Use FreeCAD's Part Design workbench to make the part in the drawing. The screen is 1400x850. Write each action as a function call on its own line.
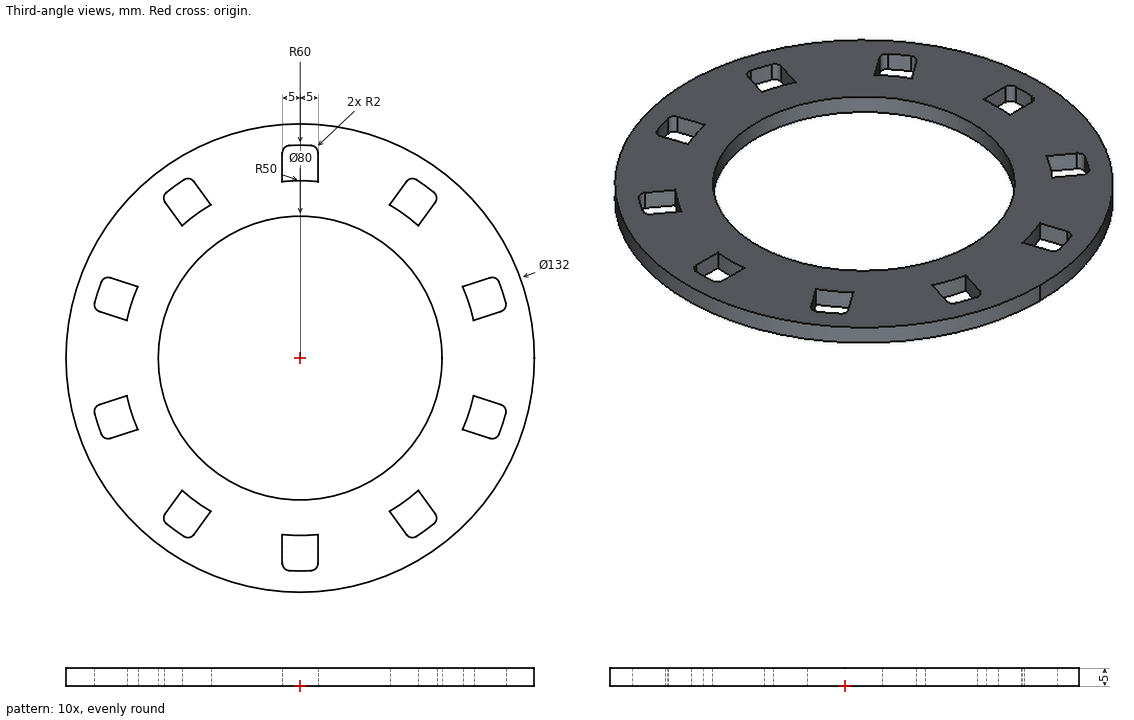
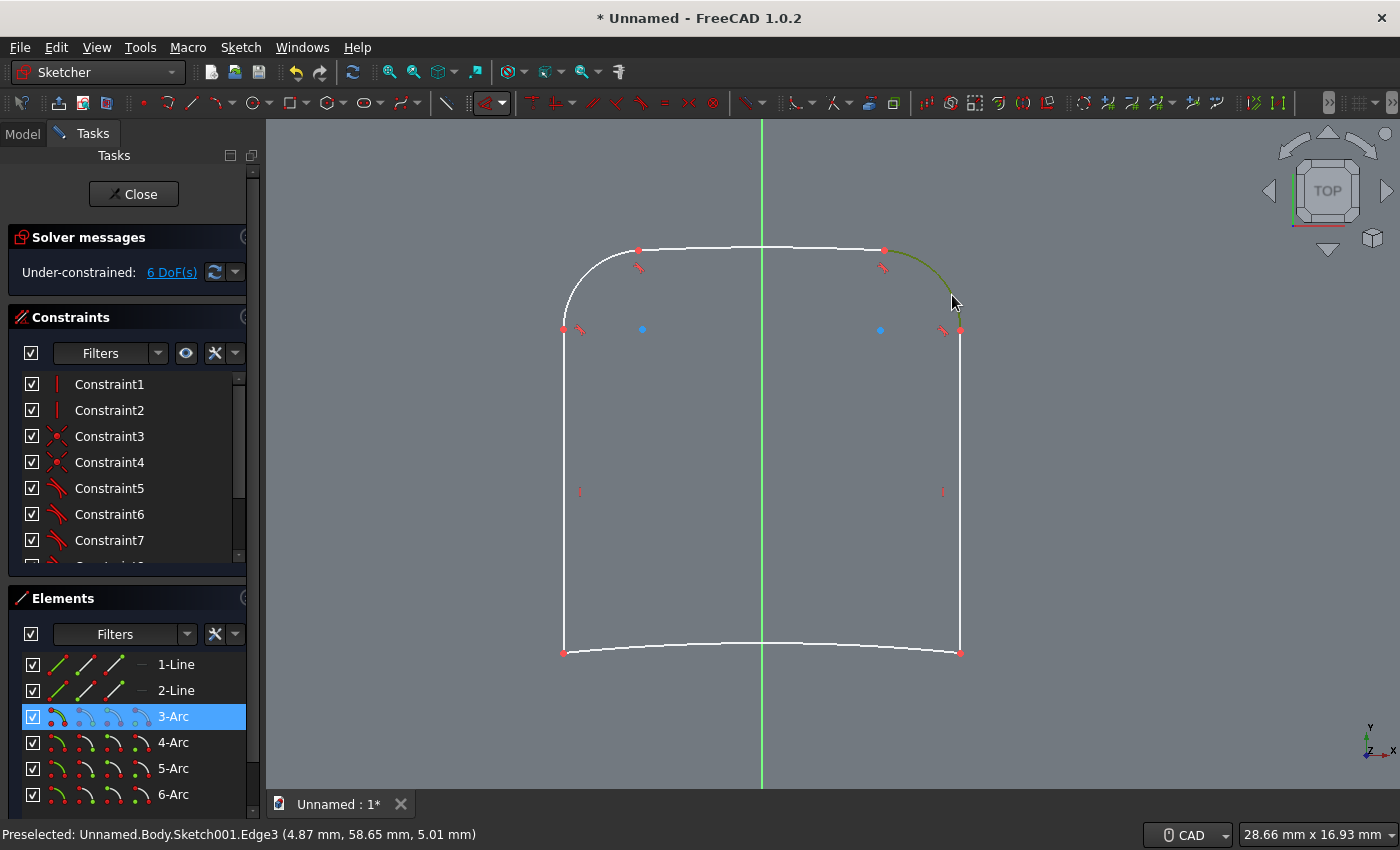
click(604, 260)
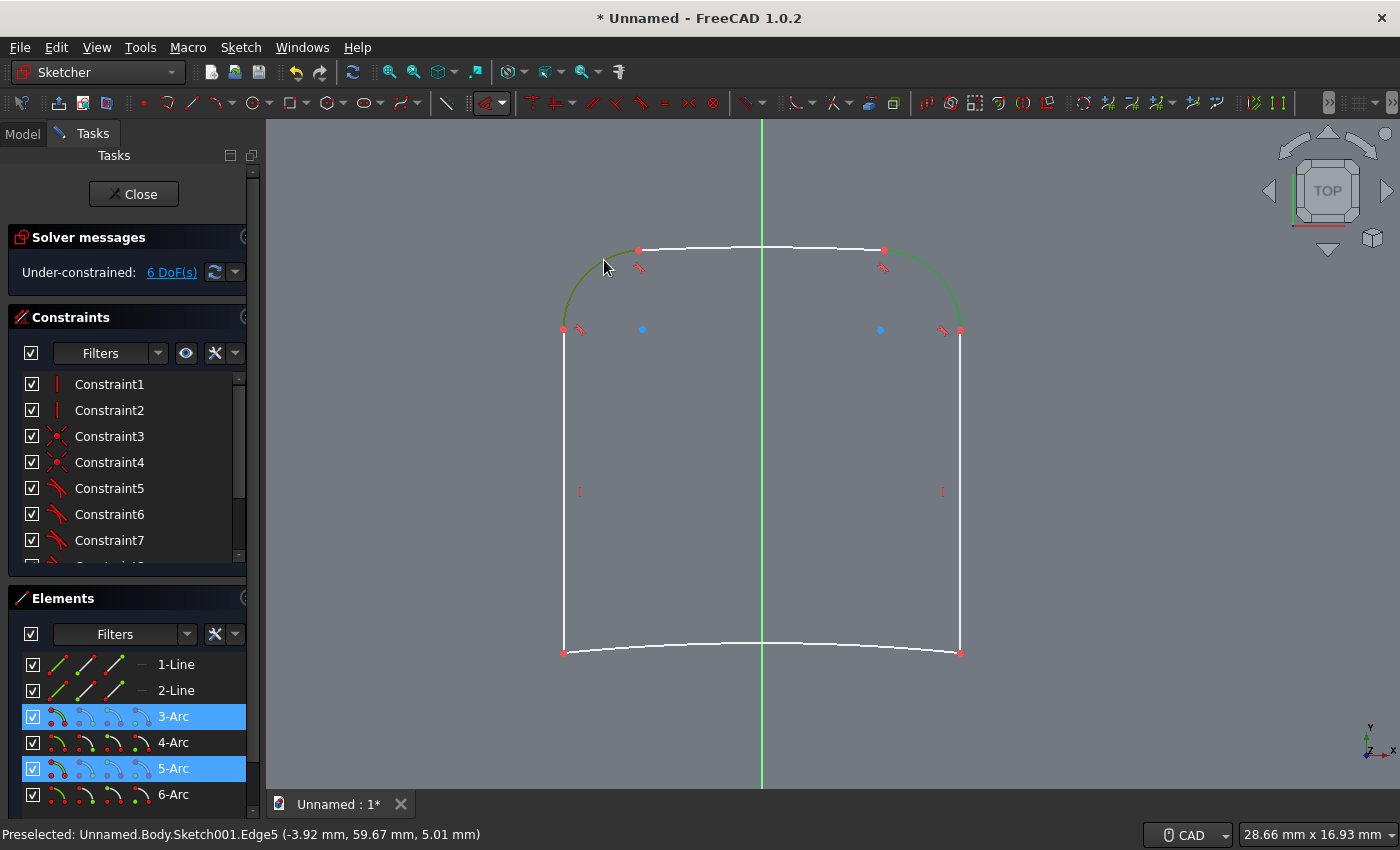
key(e)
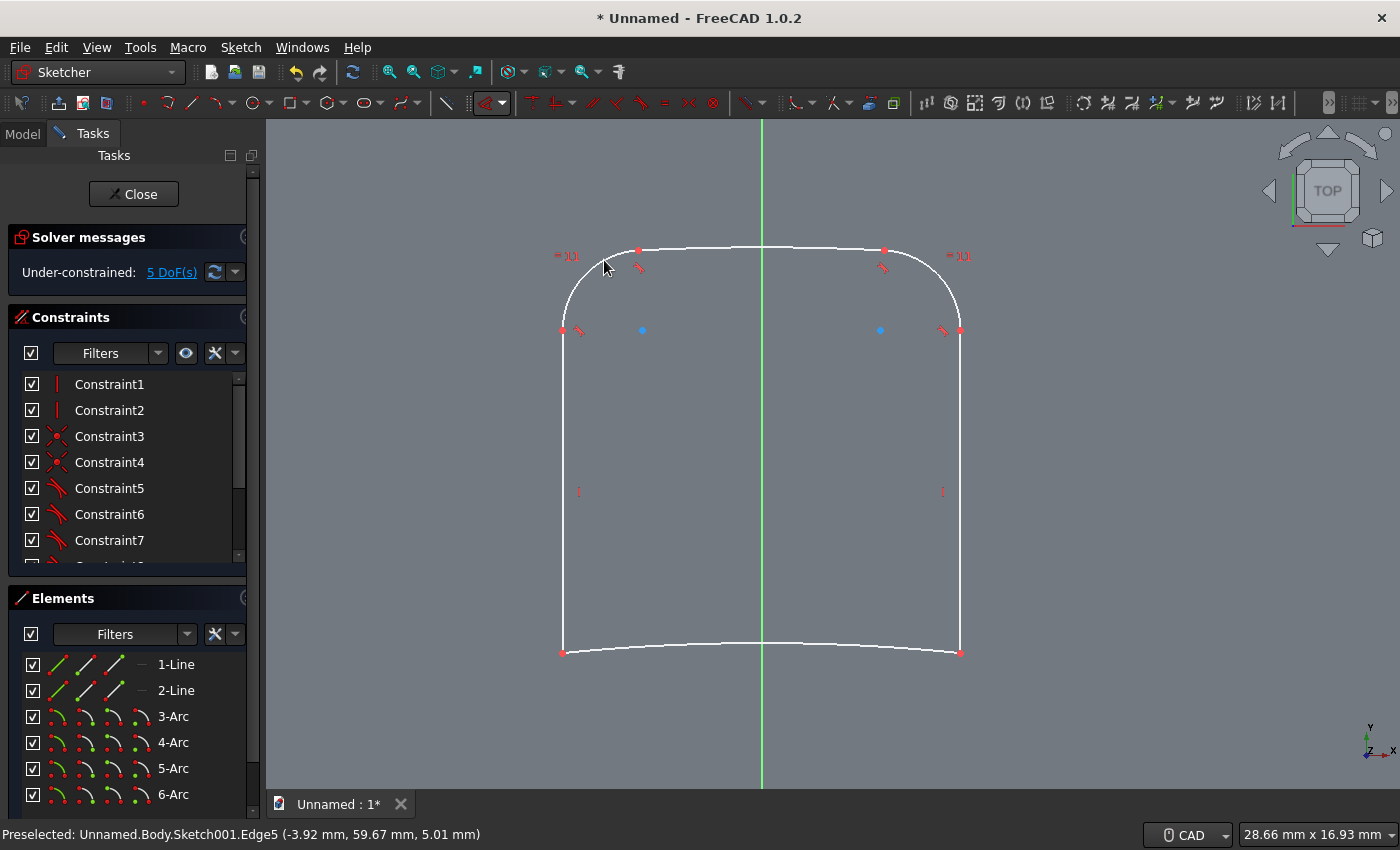
key(d)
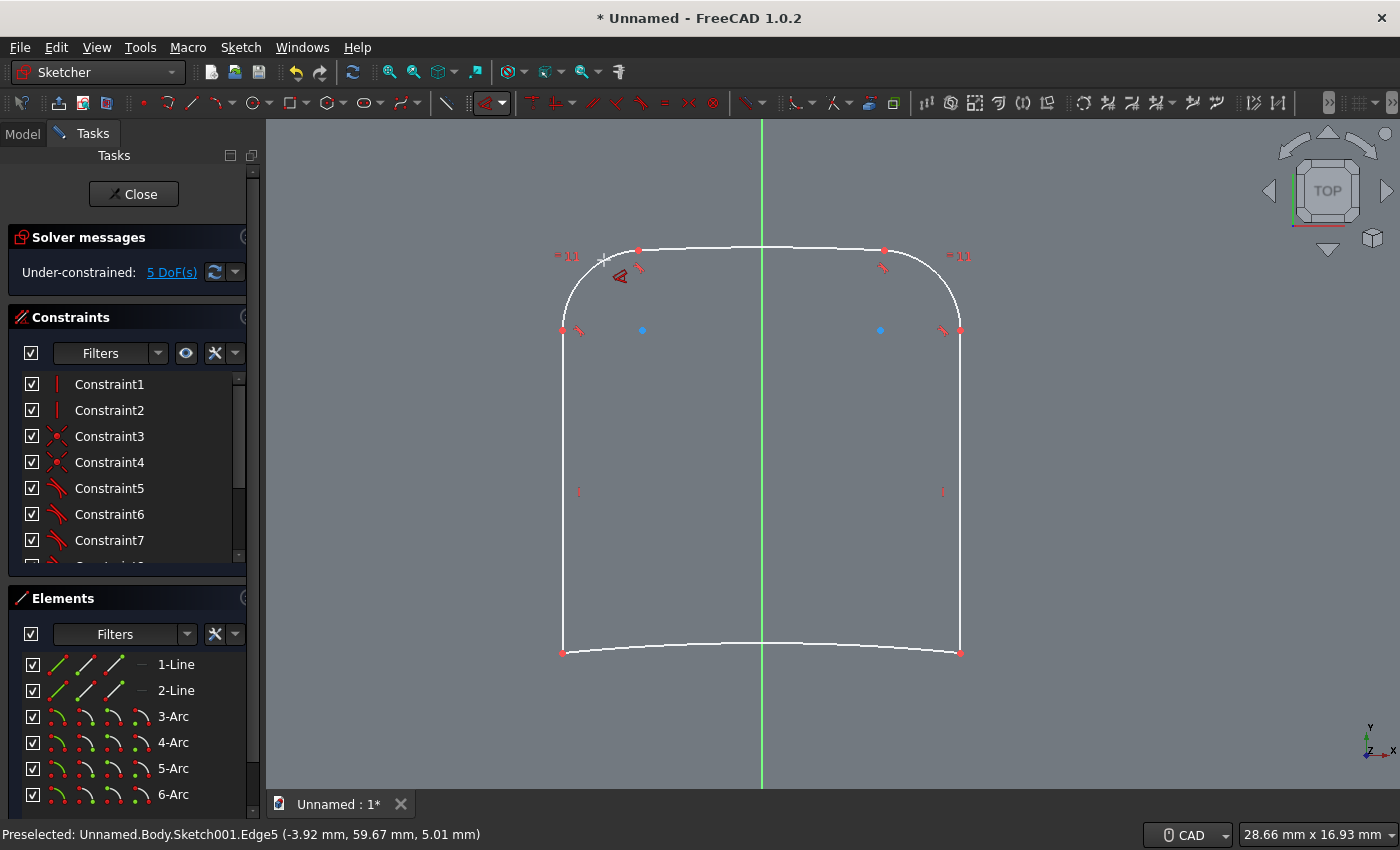
click(952, 295)
click(981, 281)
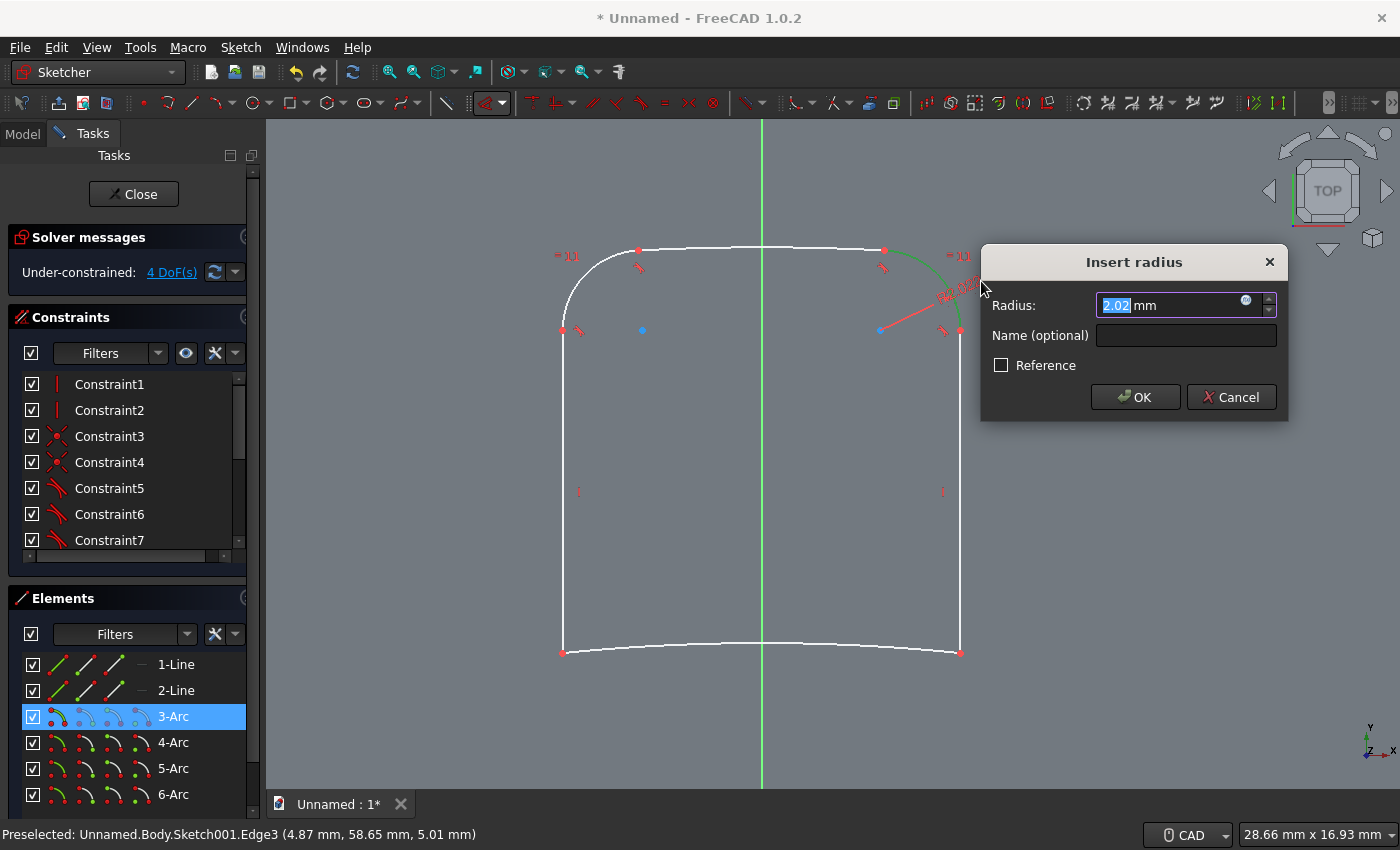
text(2)
key(Return)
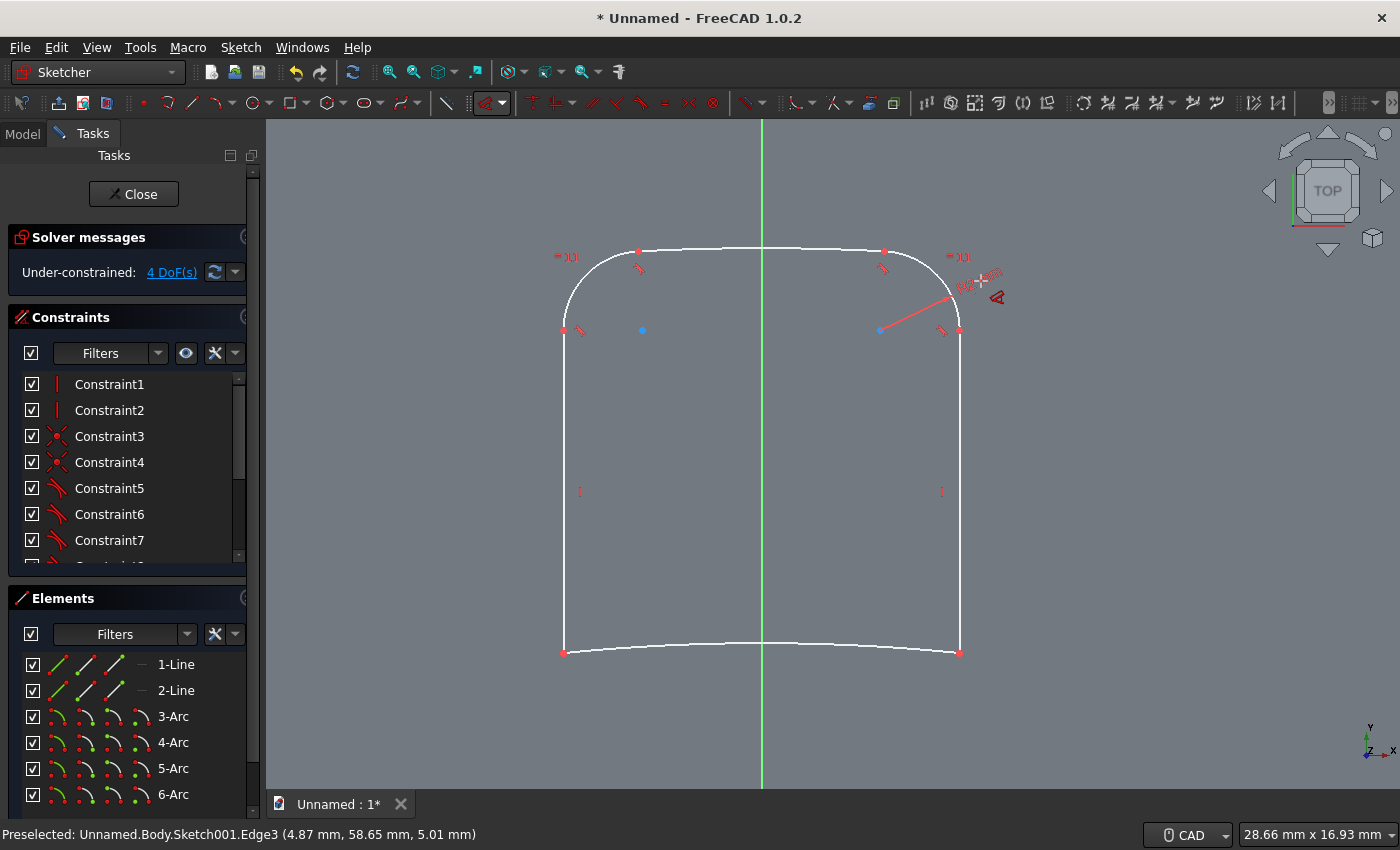
click(811, 249)
click(812, 217)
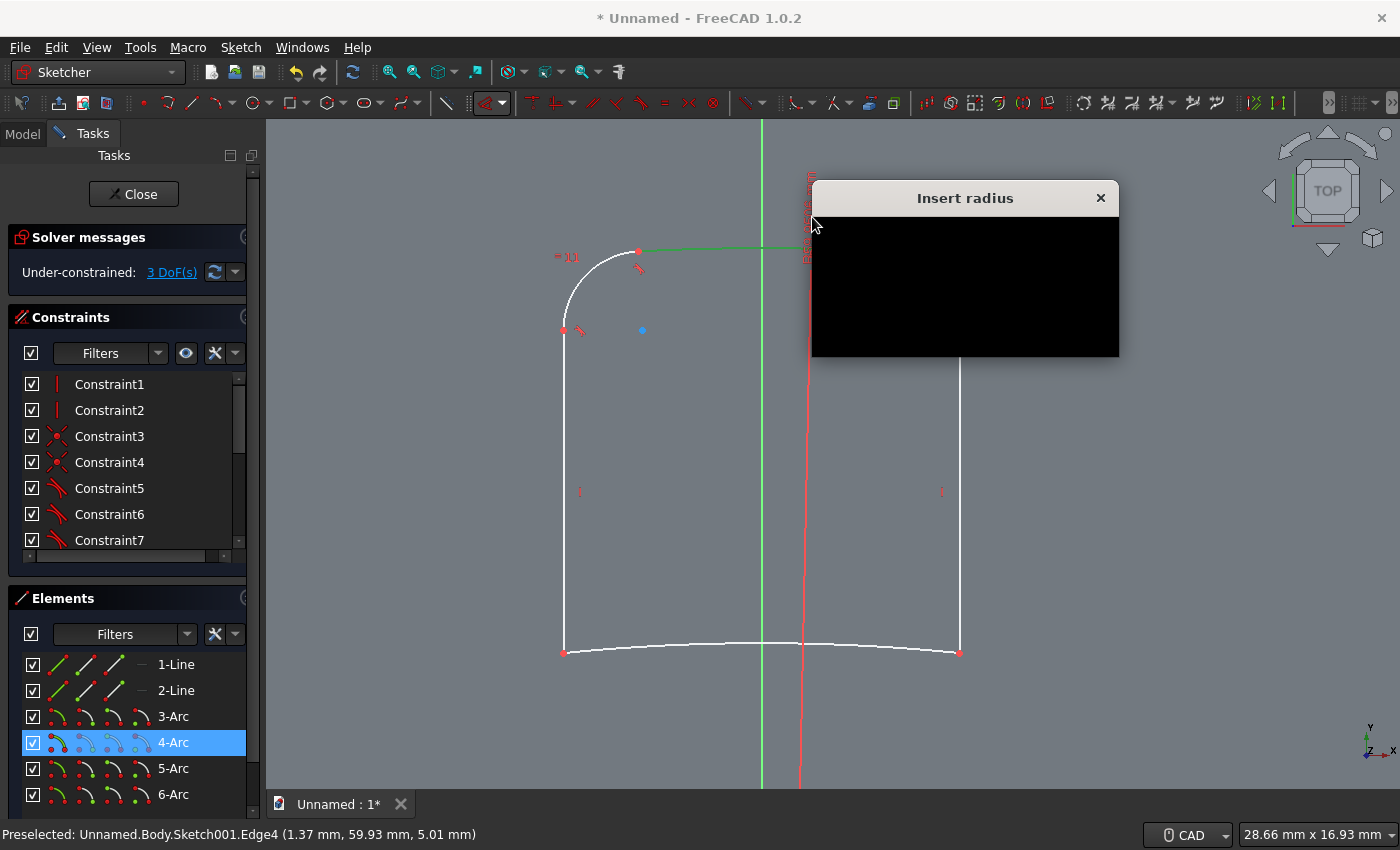
text(60)
key(Return)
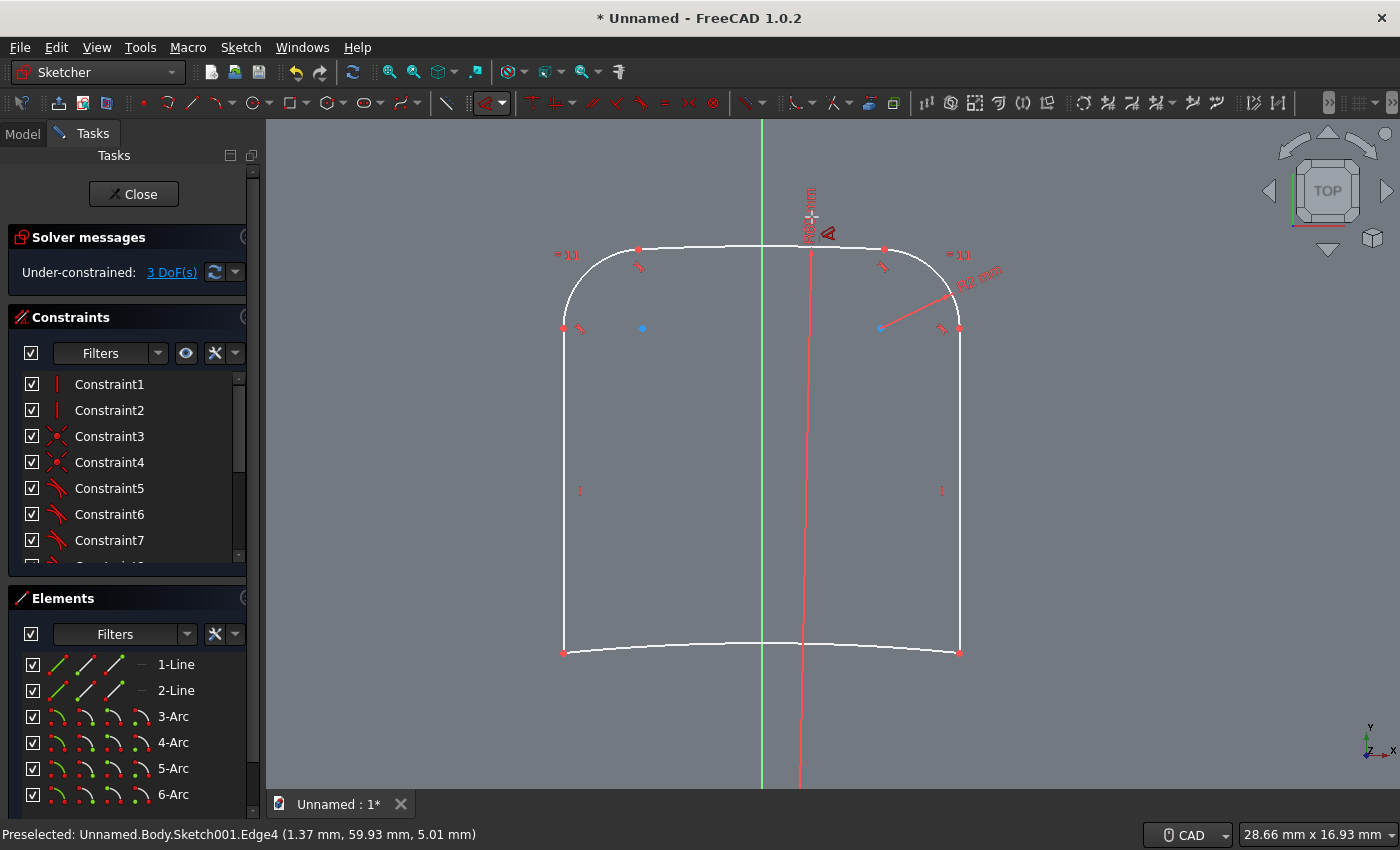
click(841, 645)
click(842, 613)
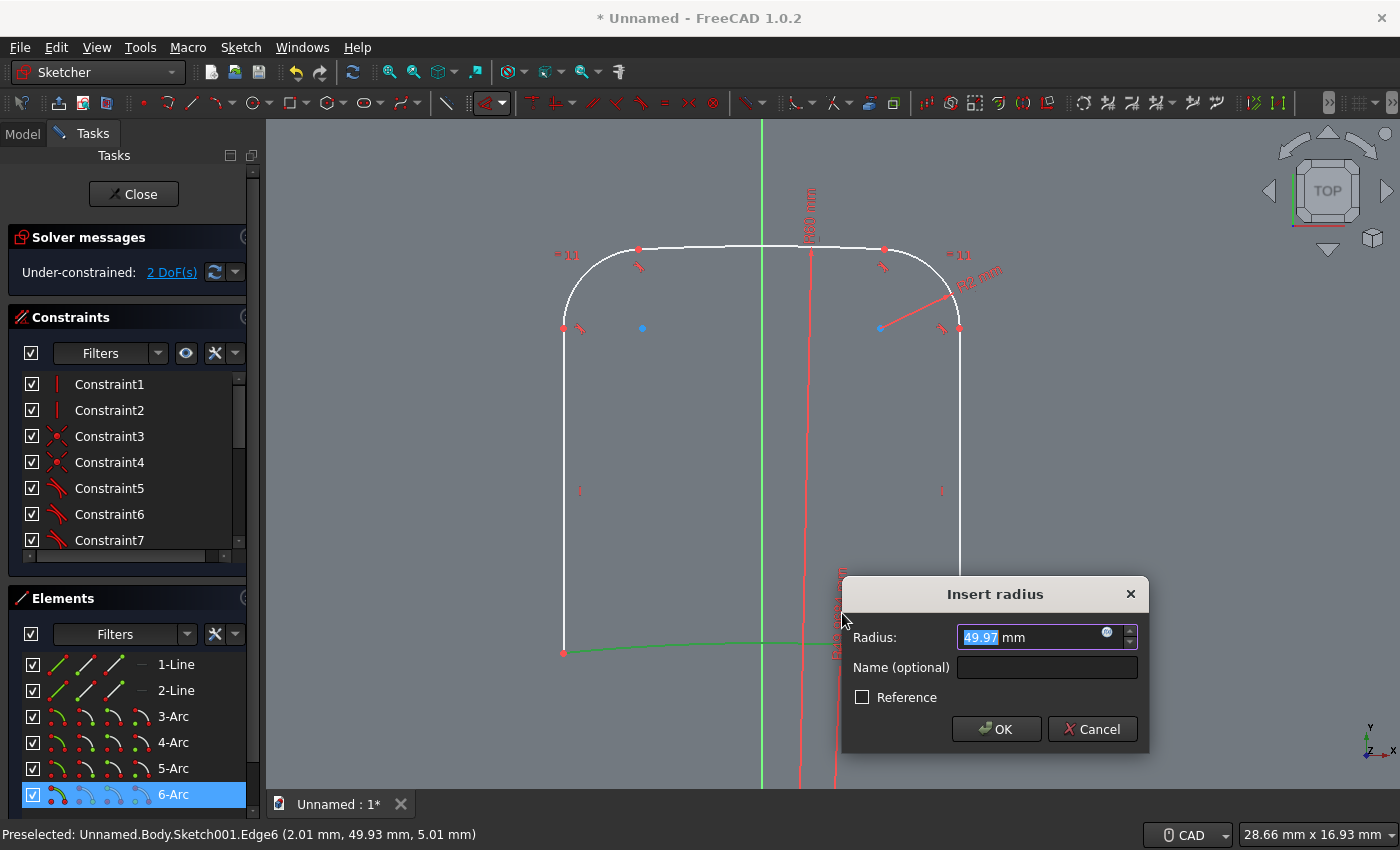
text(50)
key(Return)